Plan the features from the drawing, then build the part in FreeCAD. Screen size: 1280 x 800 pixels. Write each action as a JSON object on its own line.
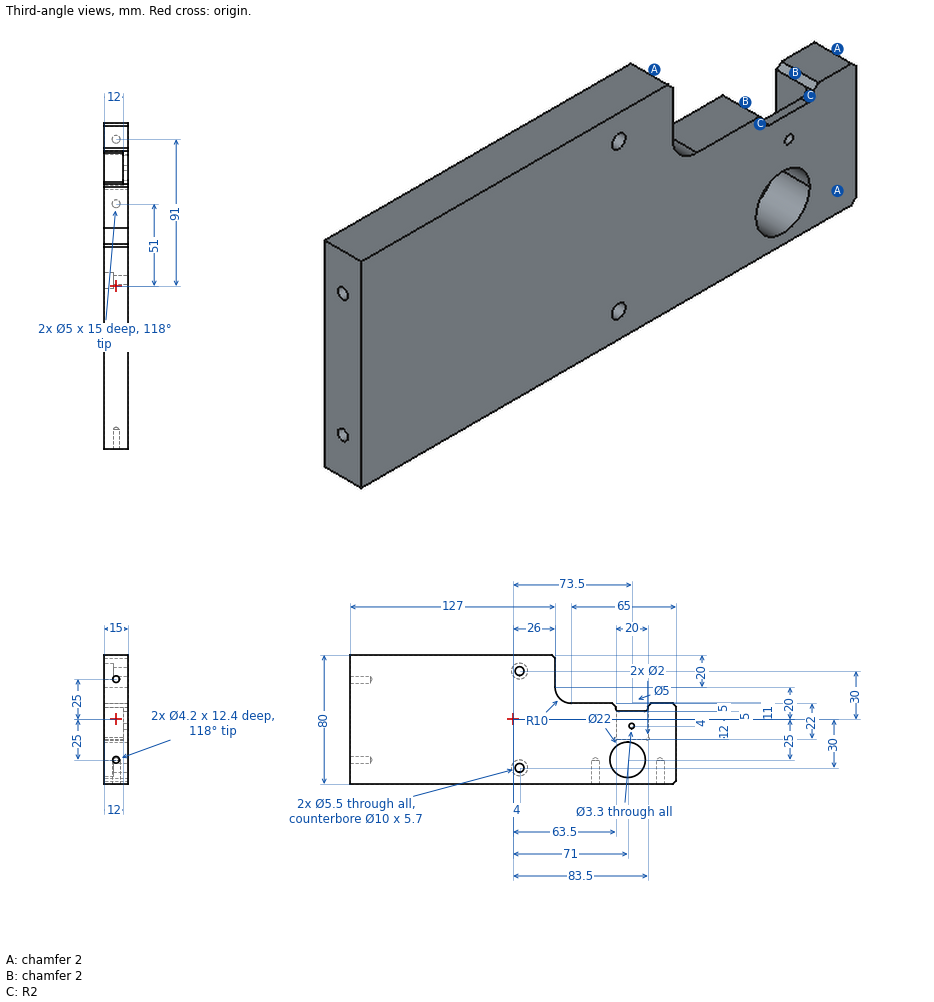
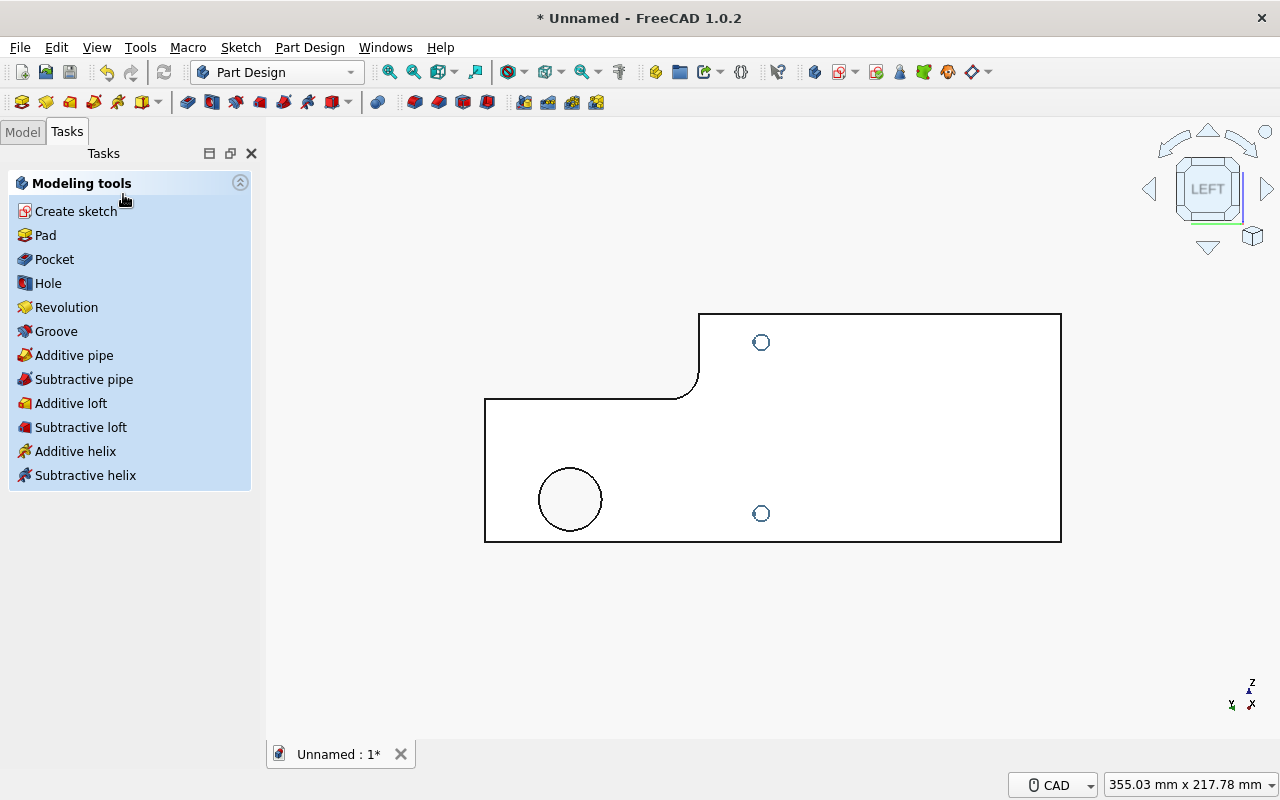
{"action": "left_click", "coordinate": [212, 102]}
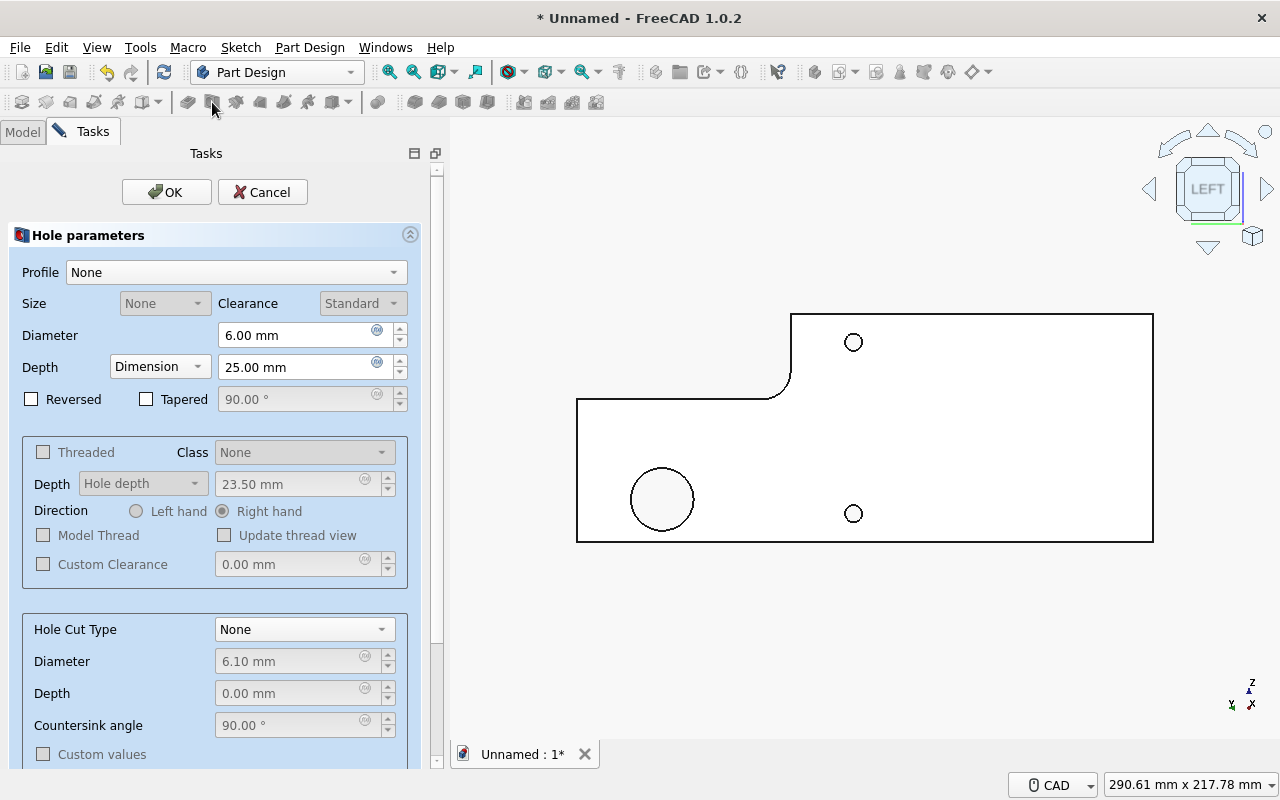
{"action": "triple_click", "coordinate": [305, 335]}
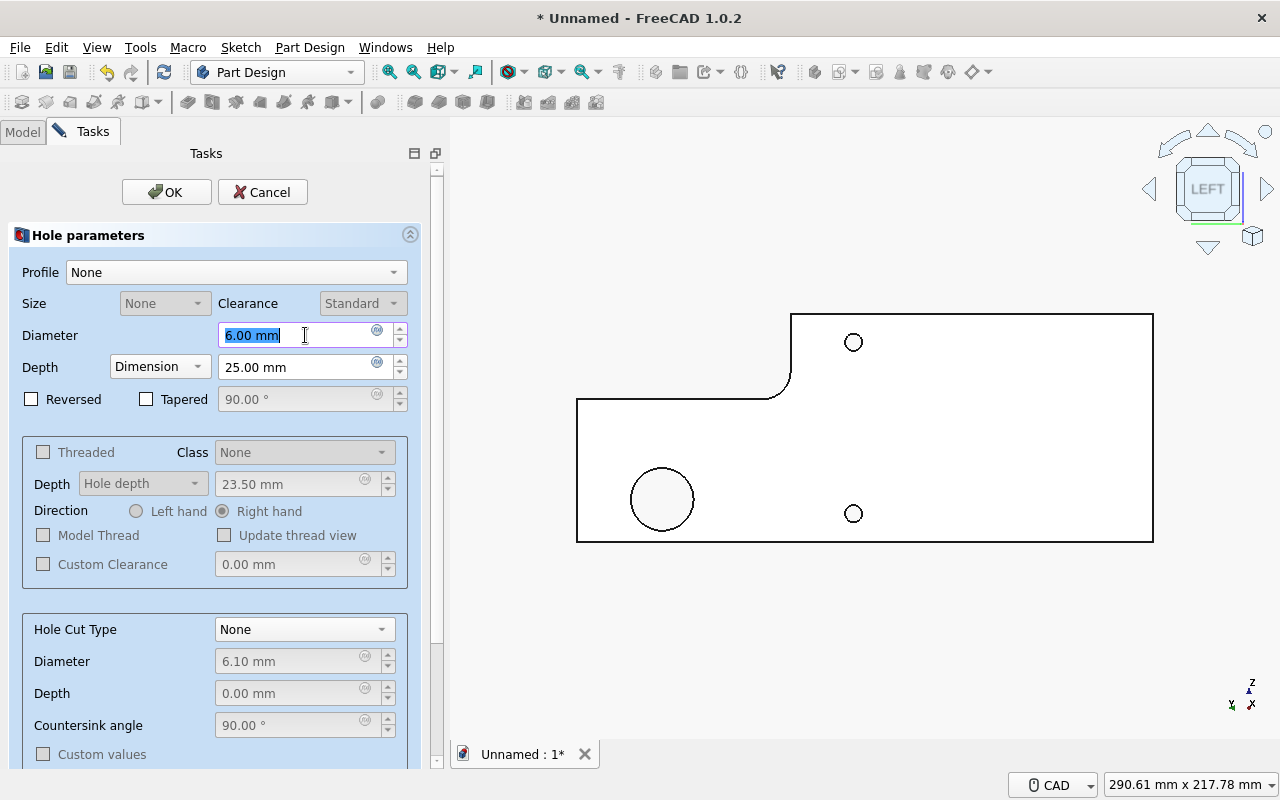
{"action": "type", "text": "5.5"}
{"action": "key", "text": "Tab"}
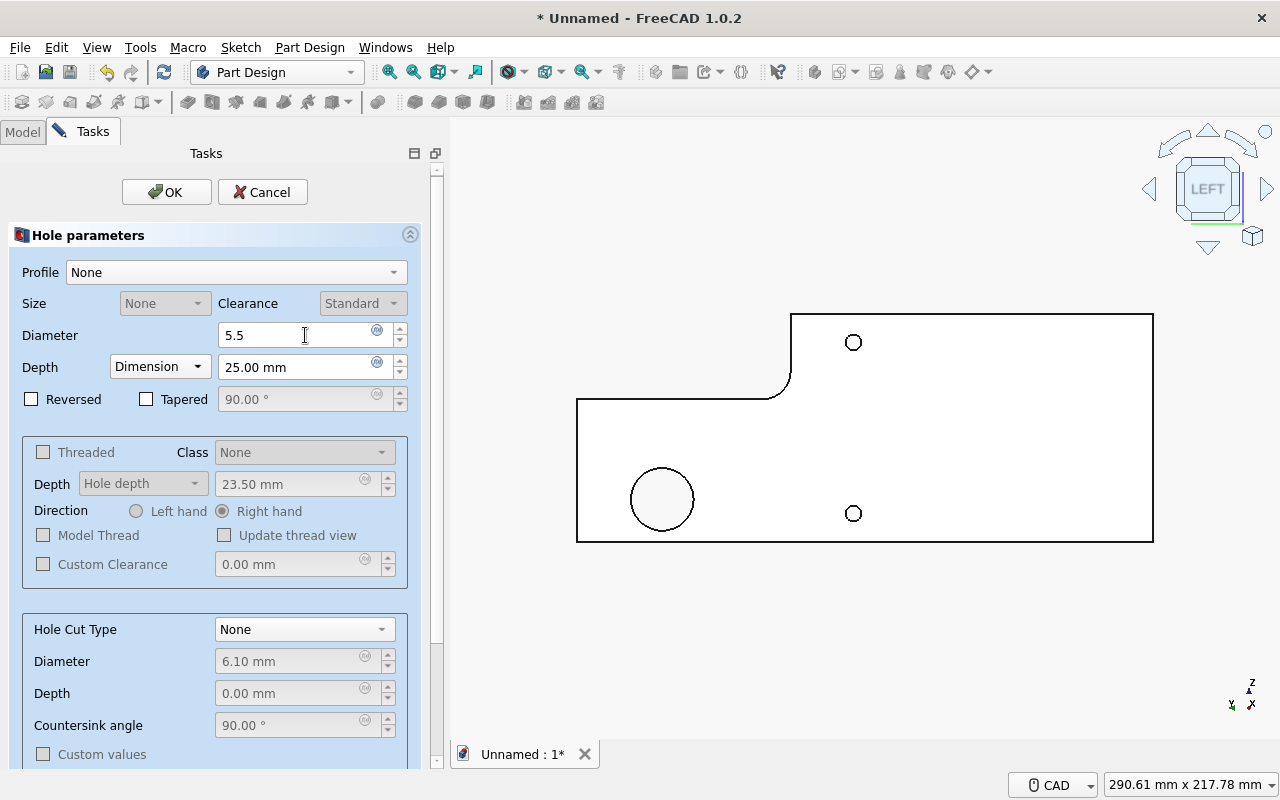
{"action": "left_click", "coordinate": [161, 366]}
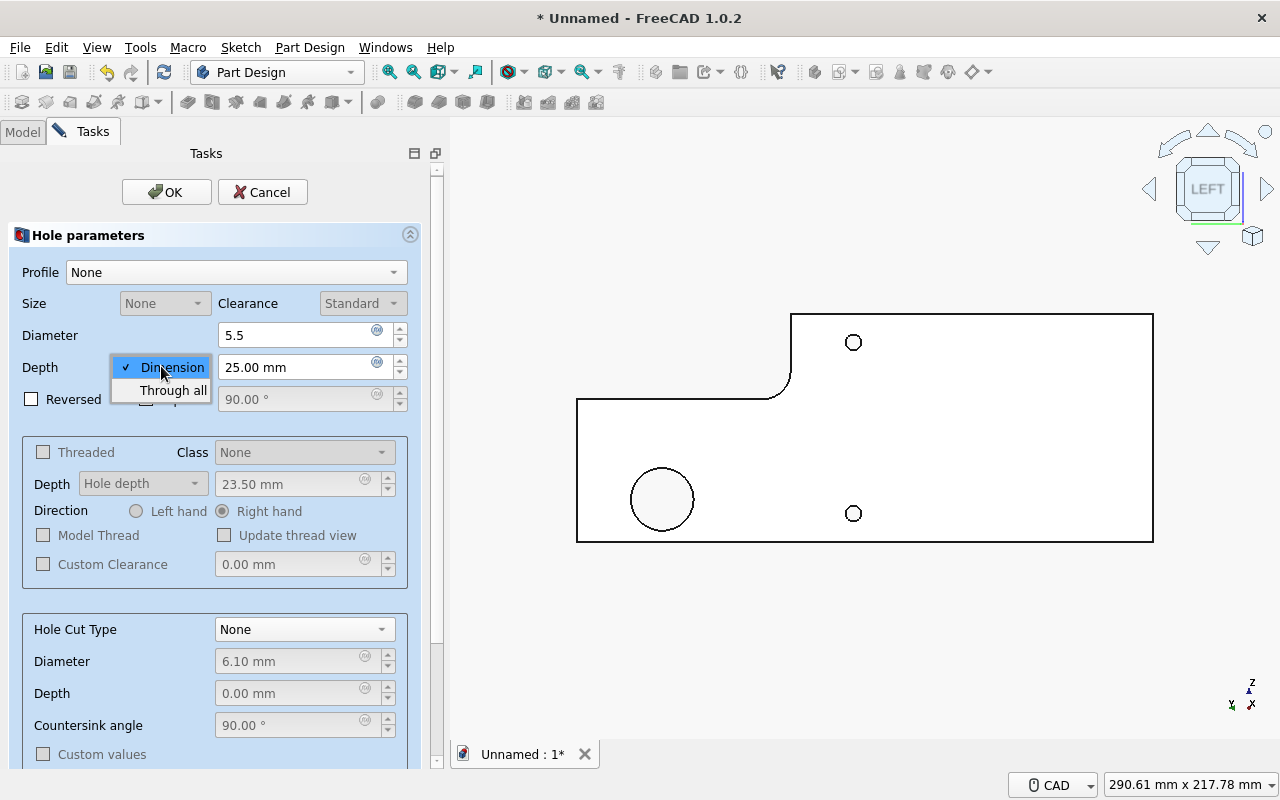
{"action": "left_click", "coordinate": [160, 390]}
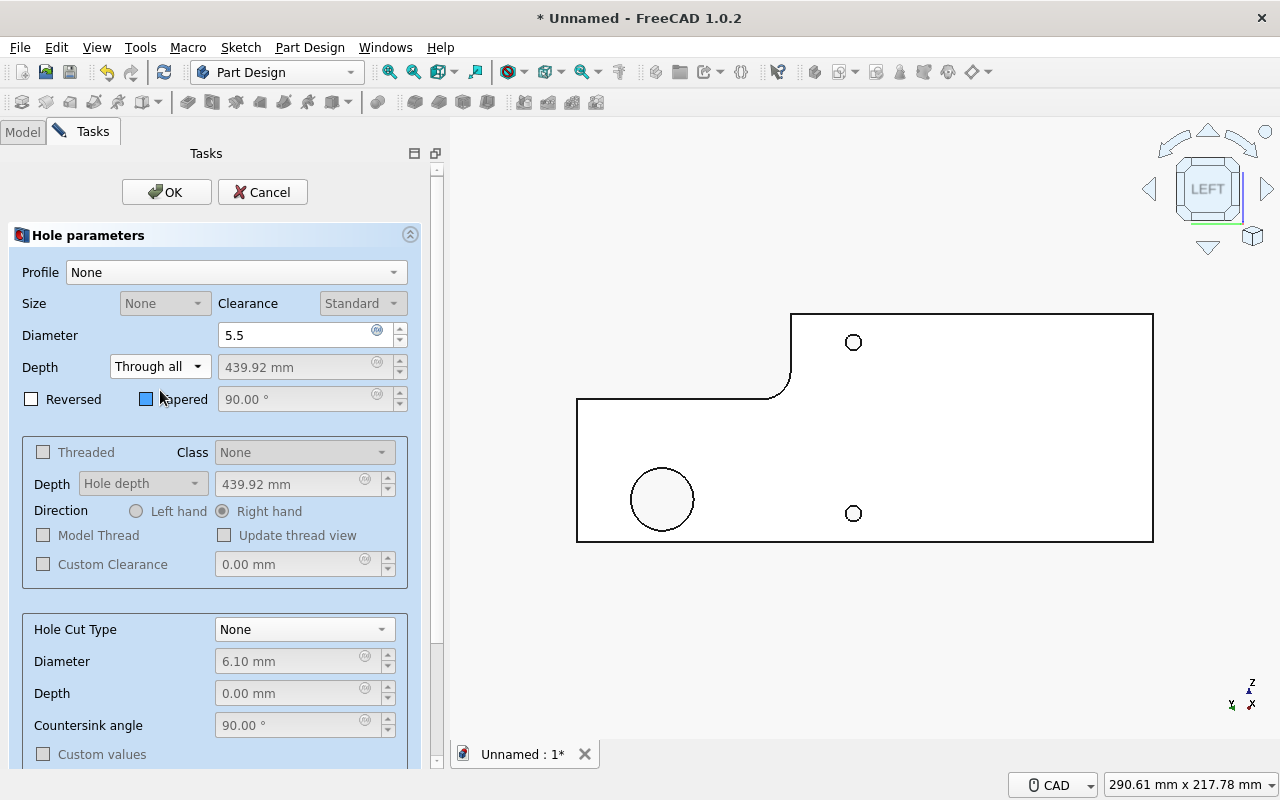
{"action": "left_click", "coordinate": [306, 630]}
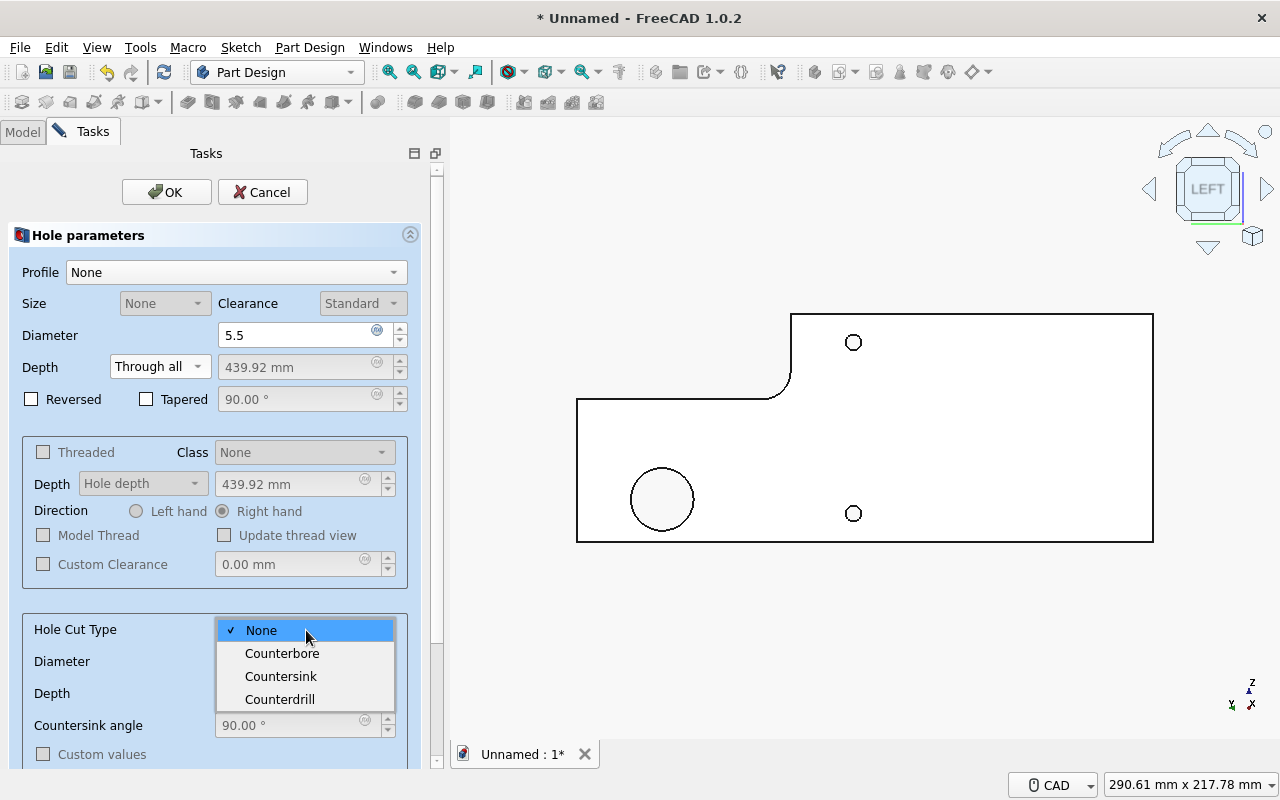
{"action": "left_click", "coordinate": [304, 654]}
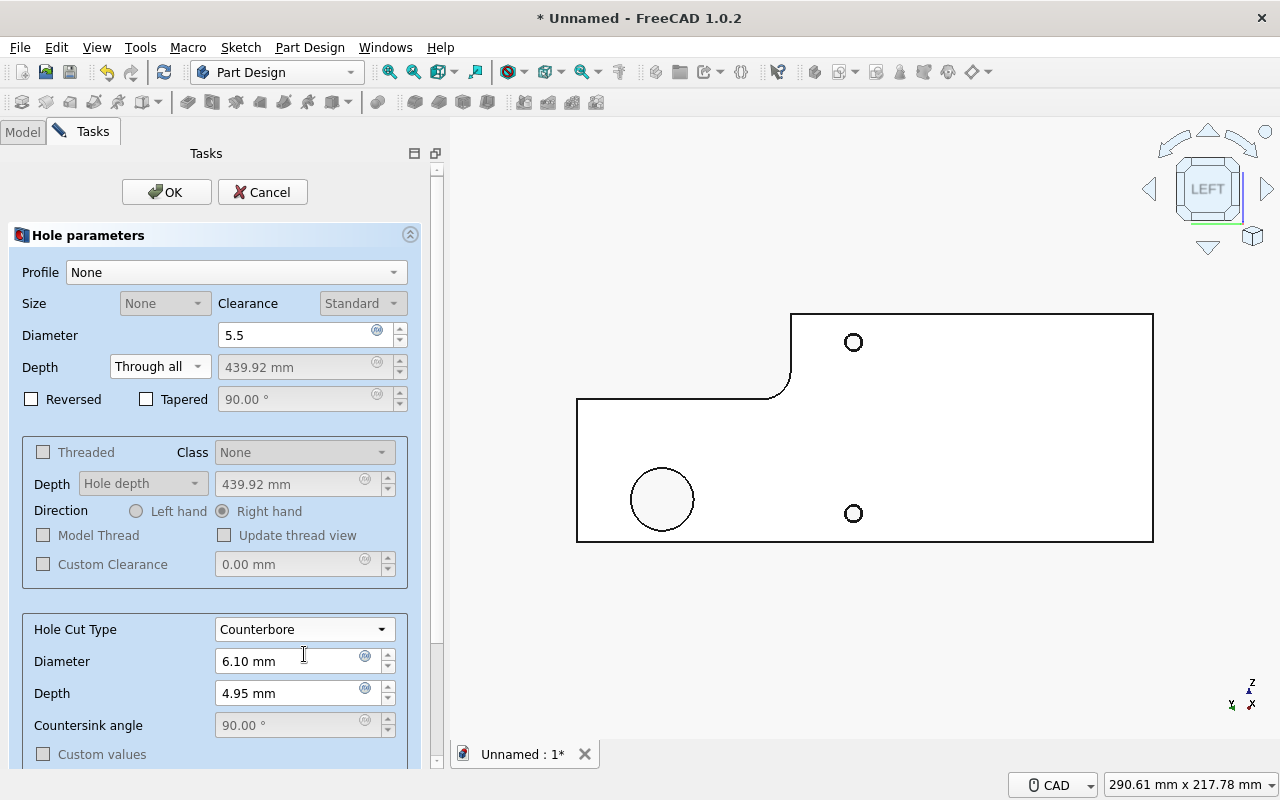
{"action": "triple_click", "coordinate": [298, 661]}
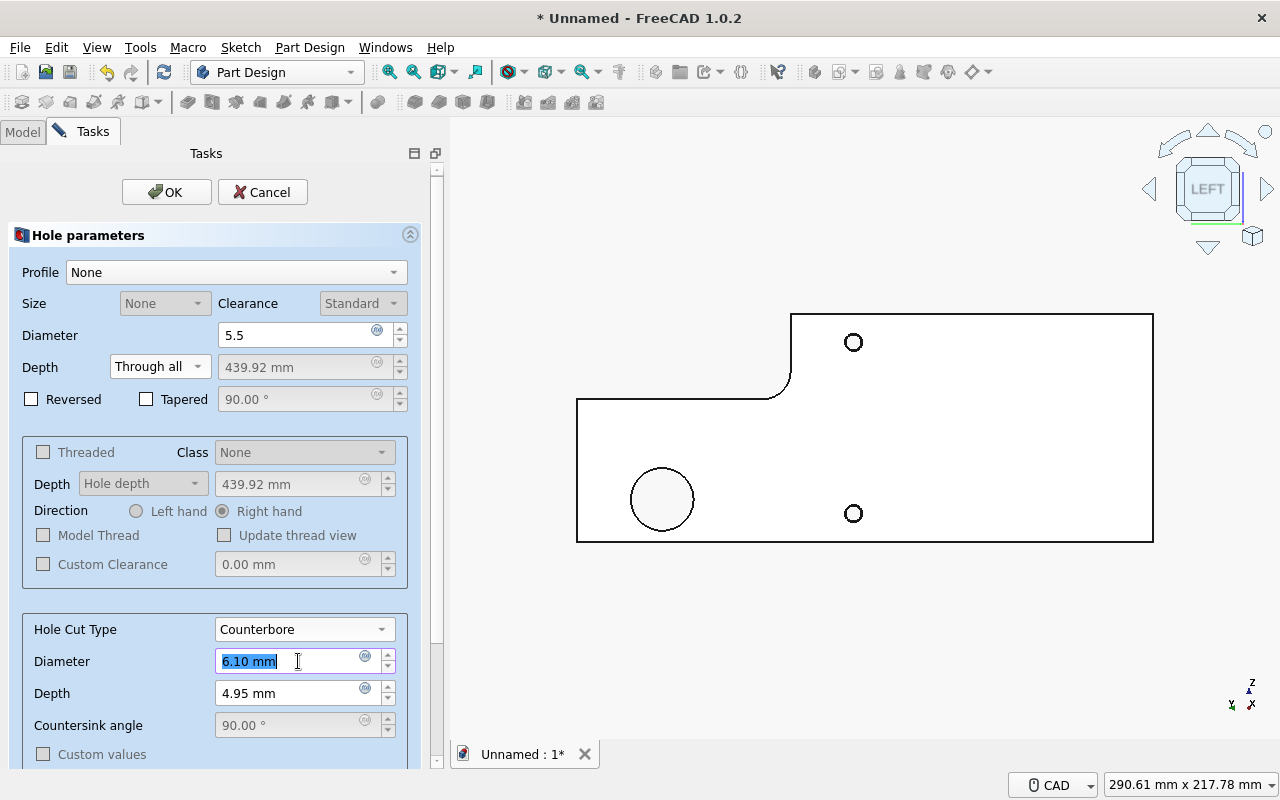
{"action": "type", "text": "10"}
{"action": "key", "text": "Tab"}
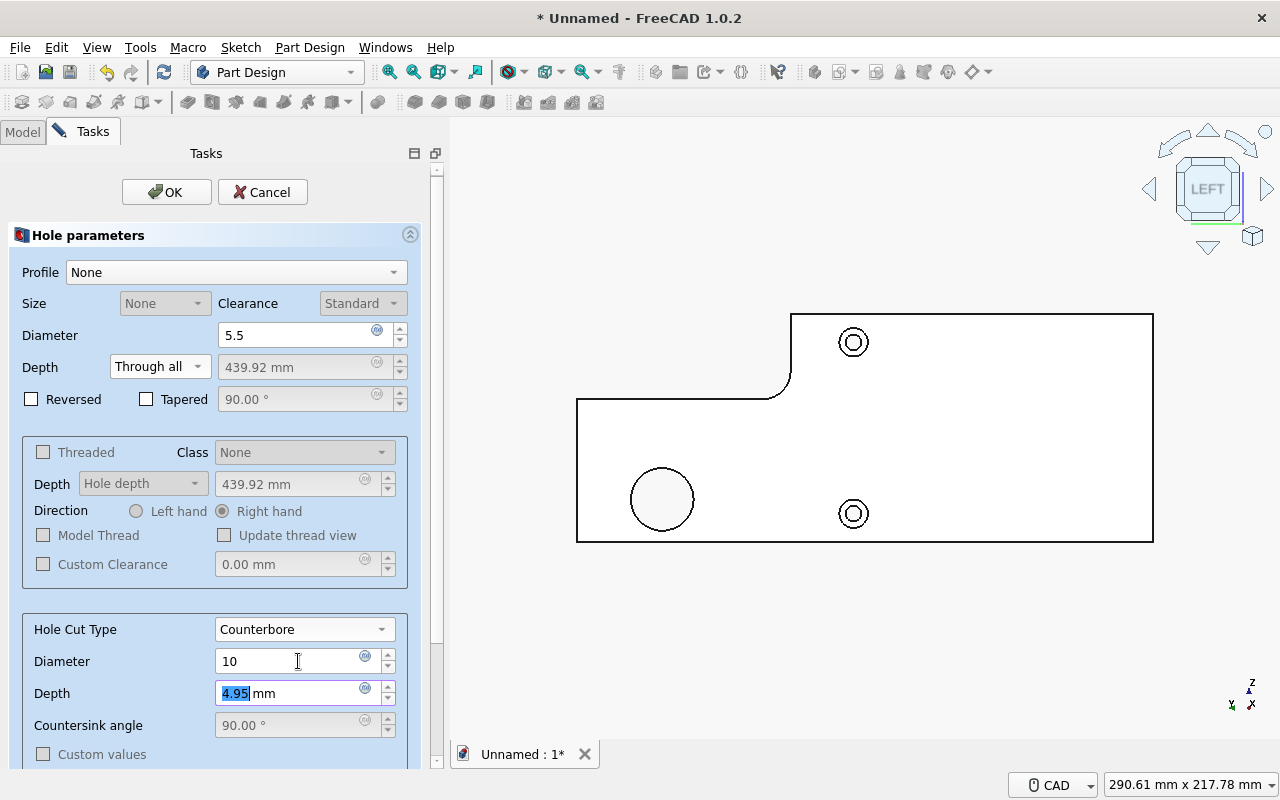
{"action": "type", "text": "5.7"}
{"action": "key", "text": "Tab"}